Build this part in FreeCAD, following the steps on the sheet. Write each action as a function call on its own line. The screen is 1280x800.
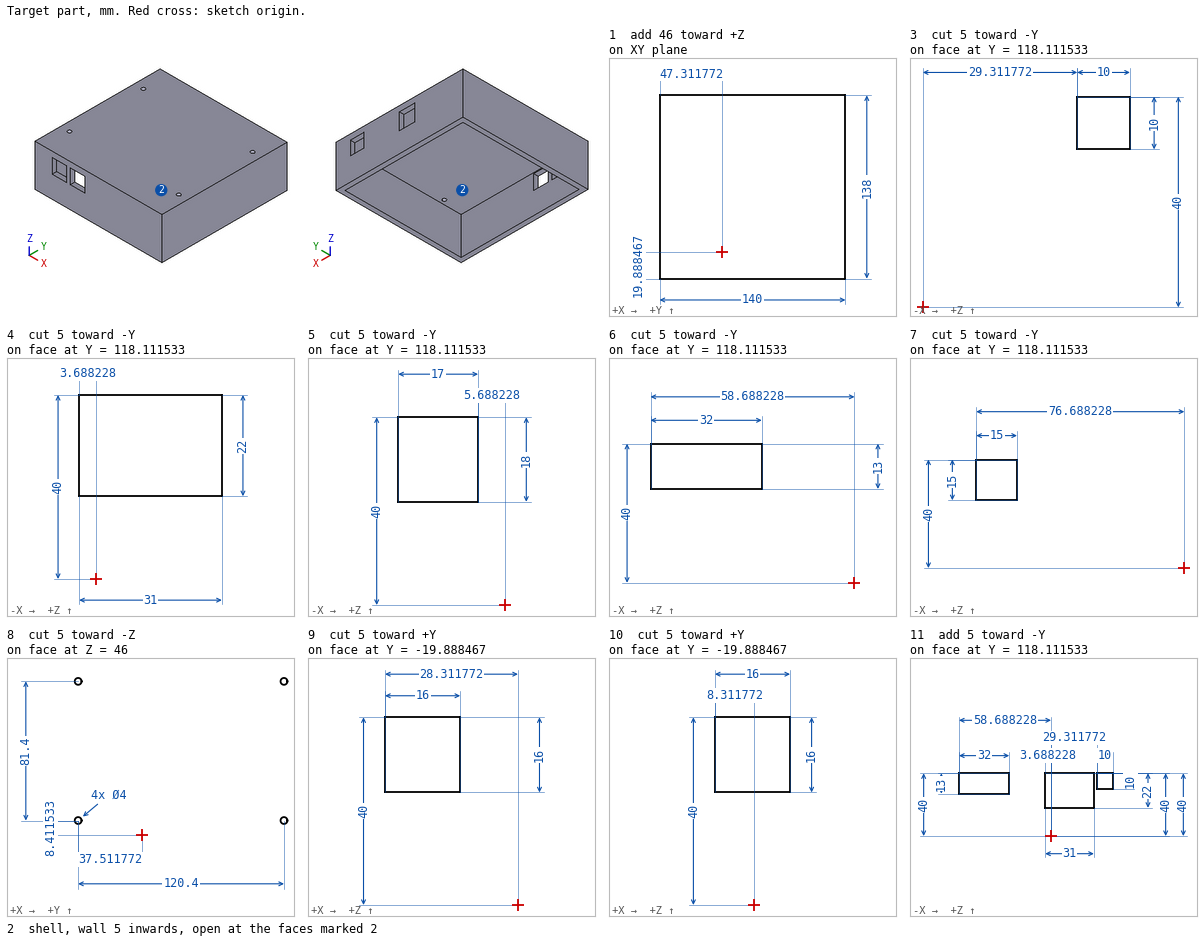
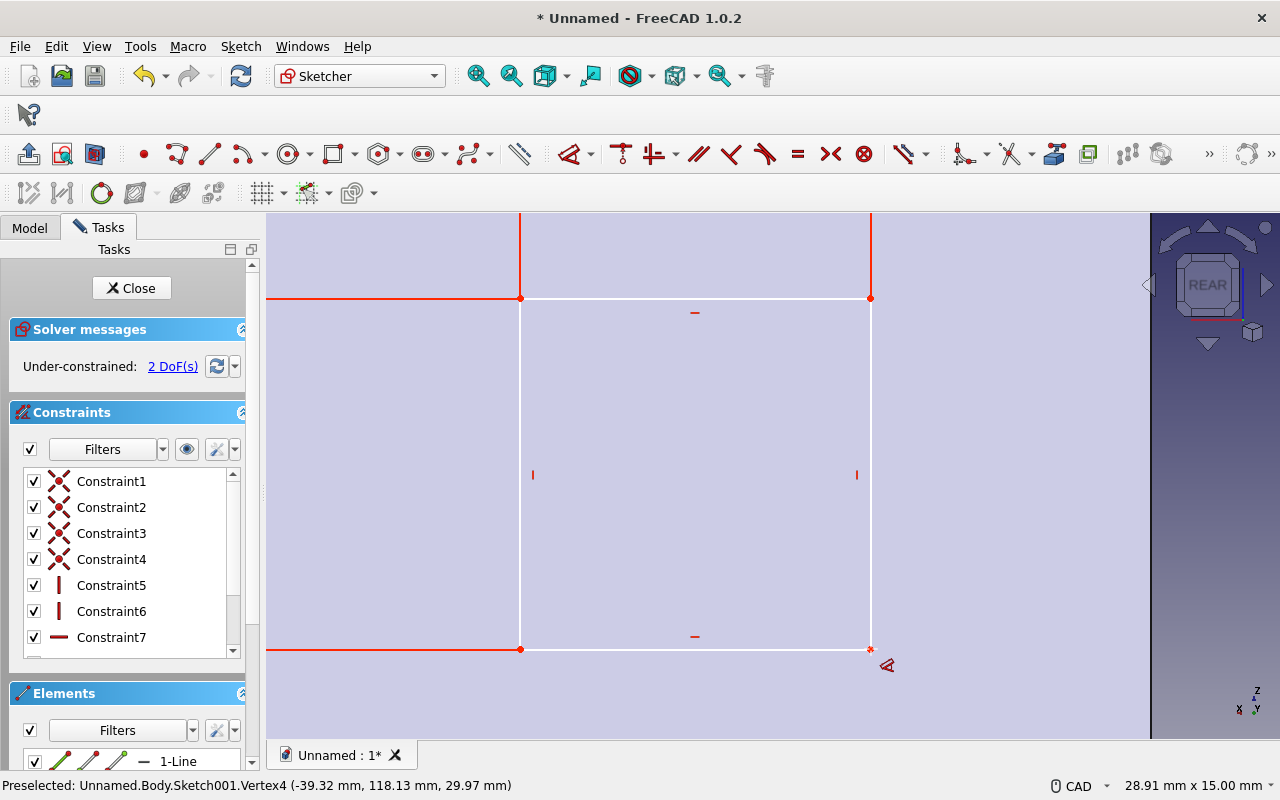
click(520, 299)
click(554, 505)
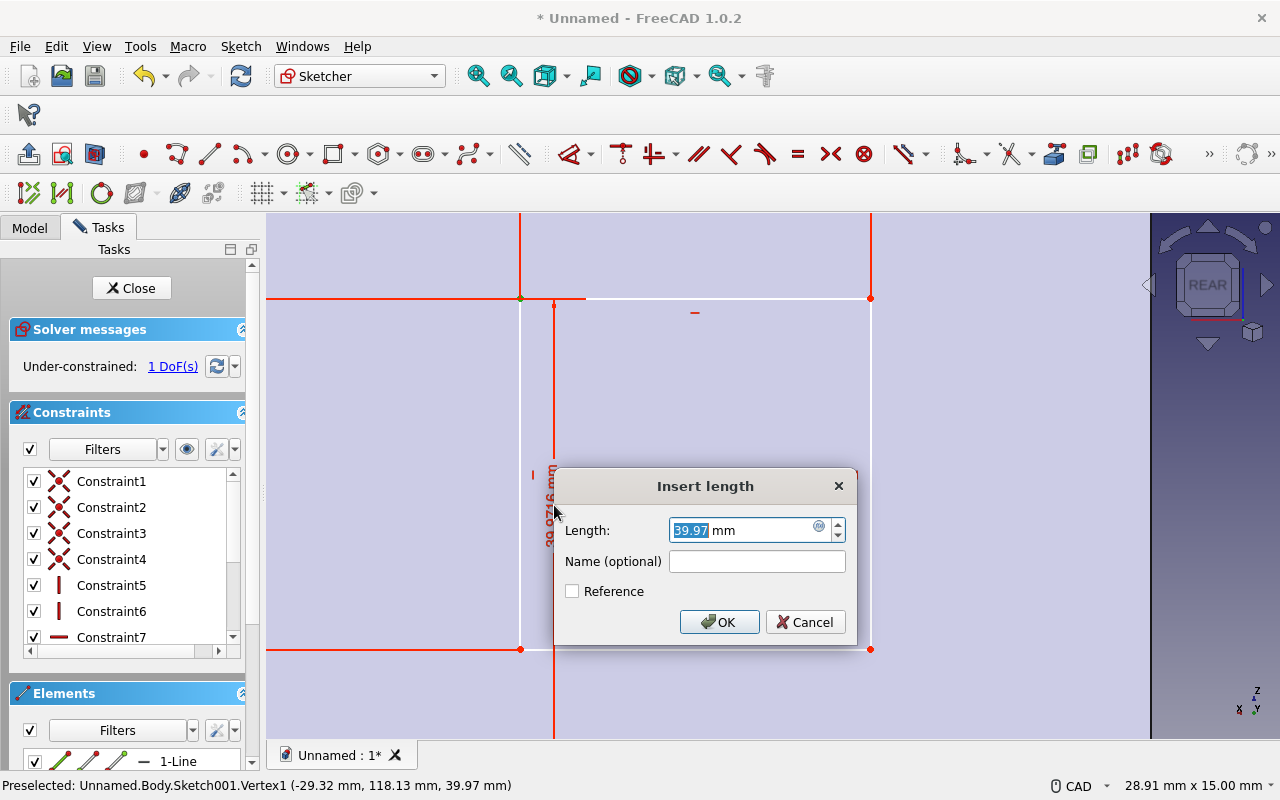
text(40)
key(Return)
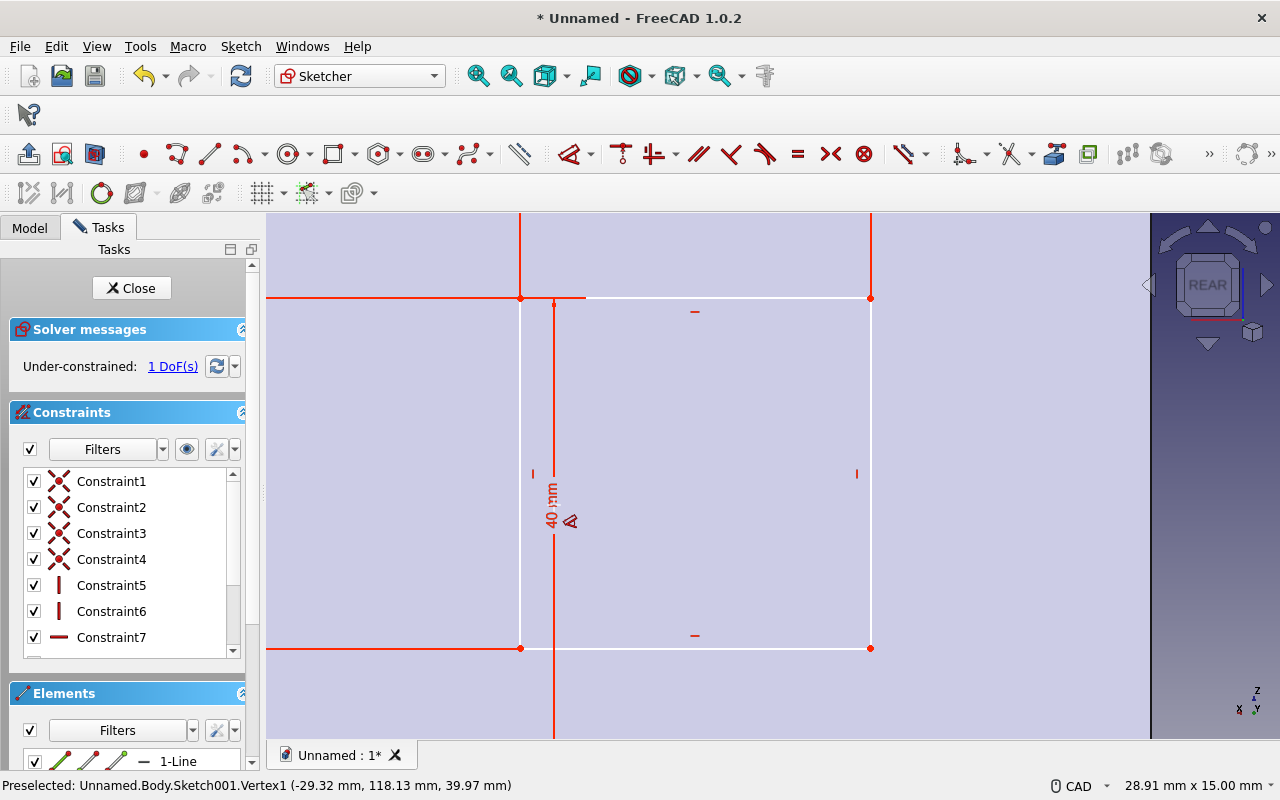
click(520, 298)
click(407, 264)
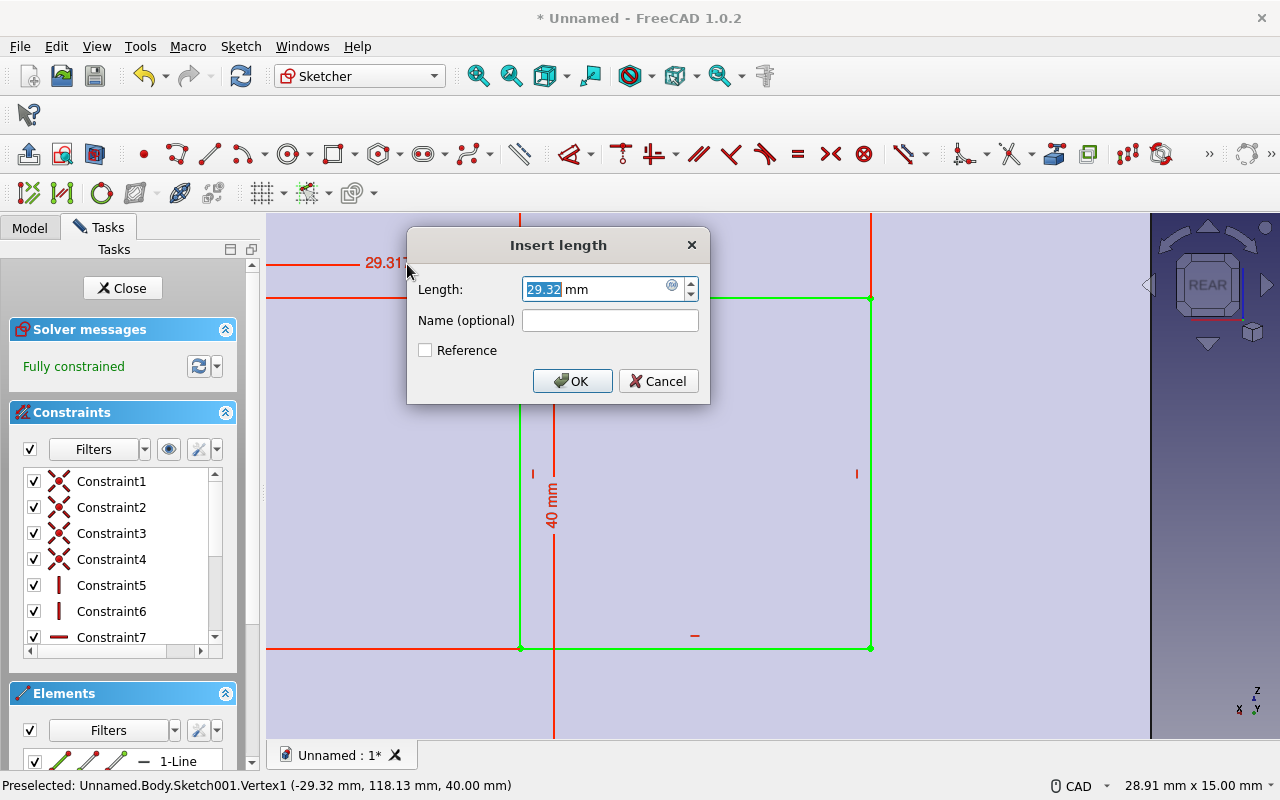
text(29.311772)
key(Return)
key(Escape)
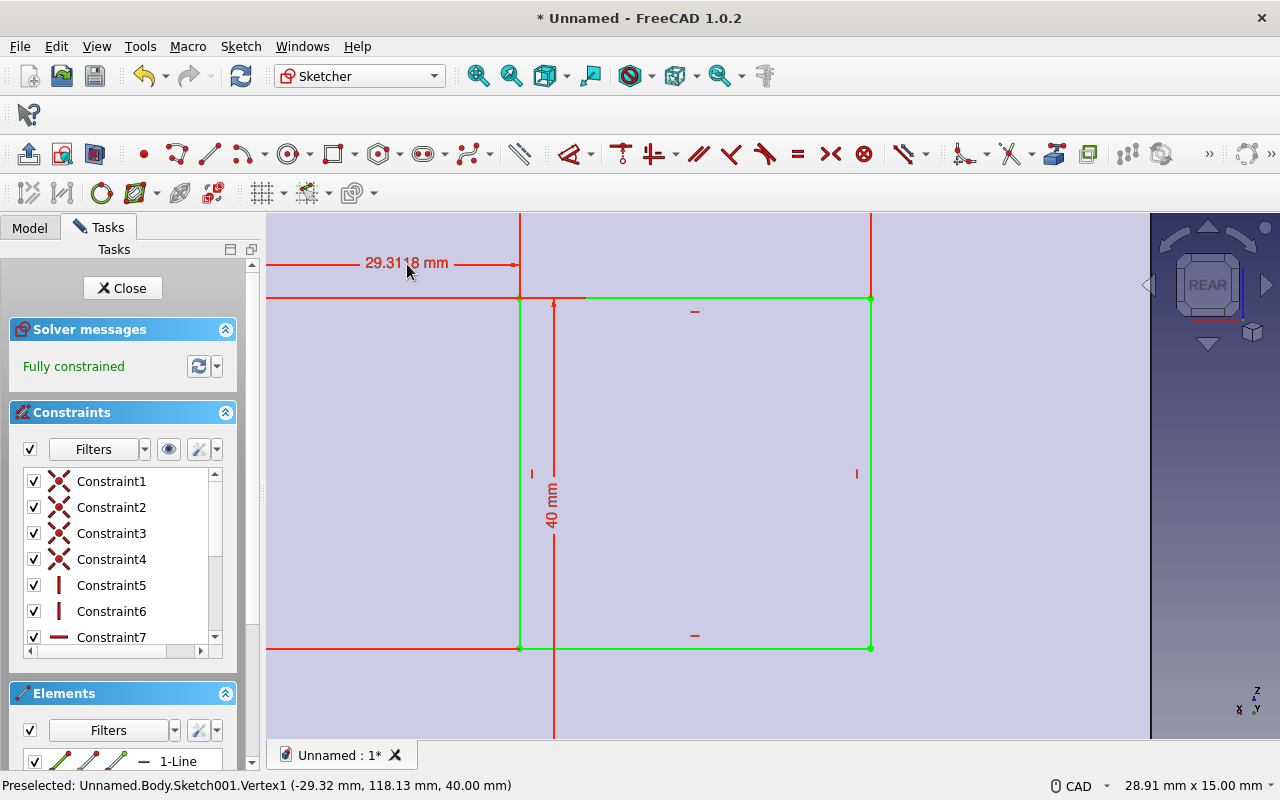
click(123, 288)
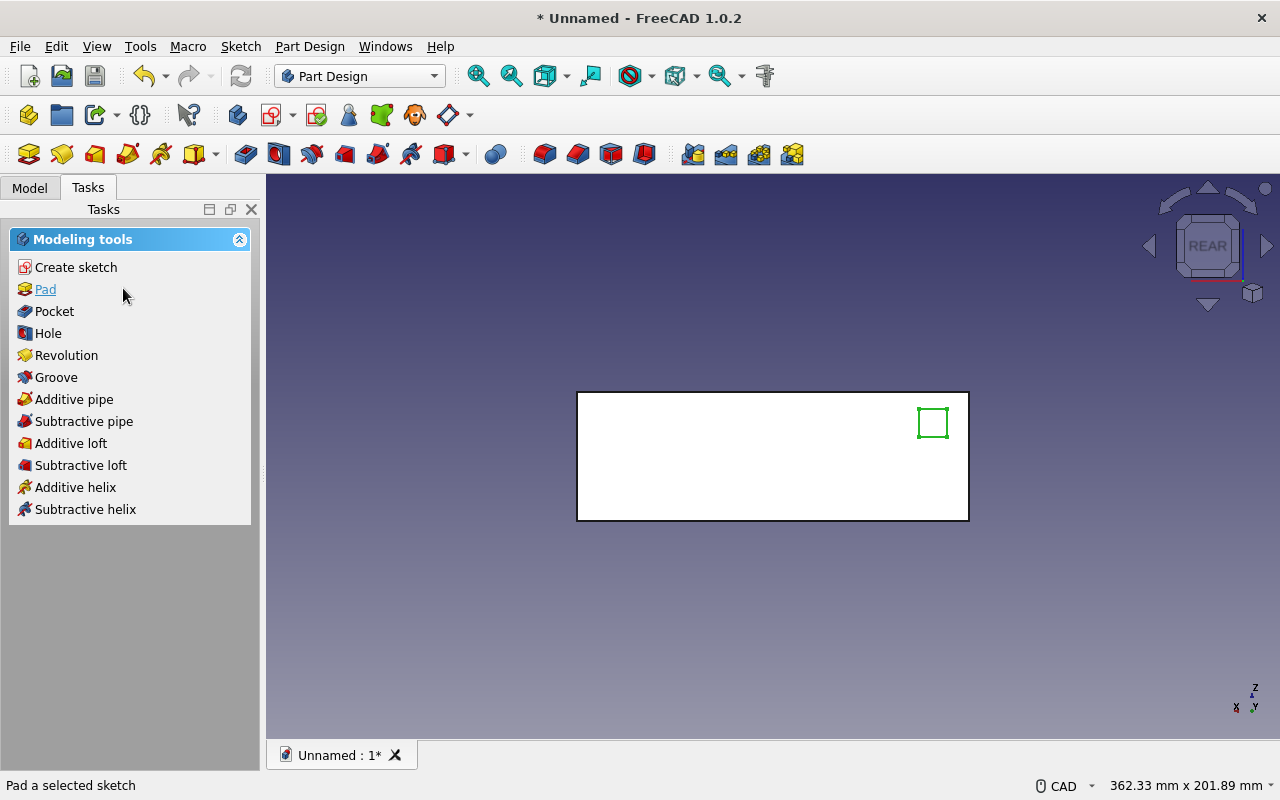
click(246, 154)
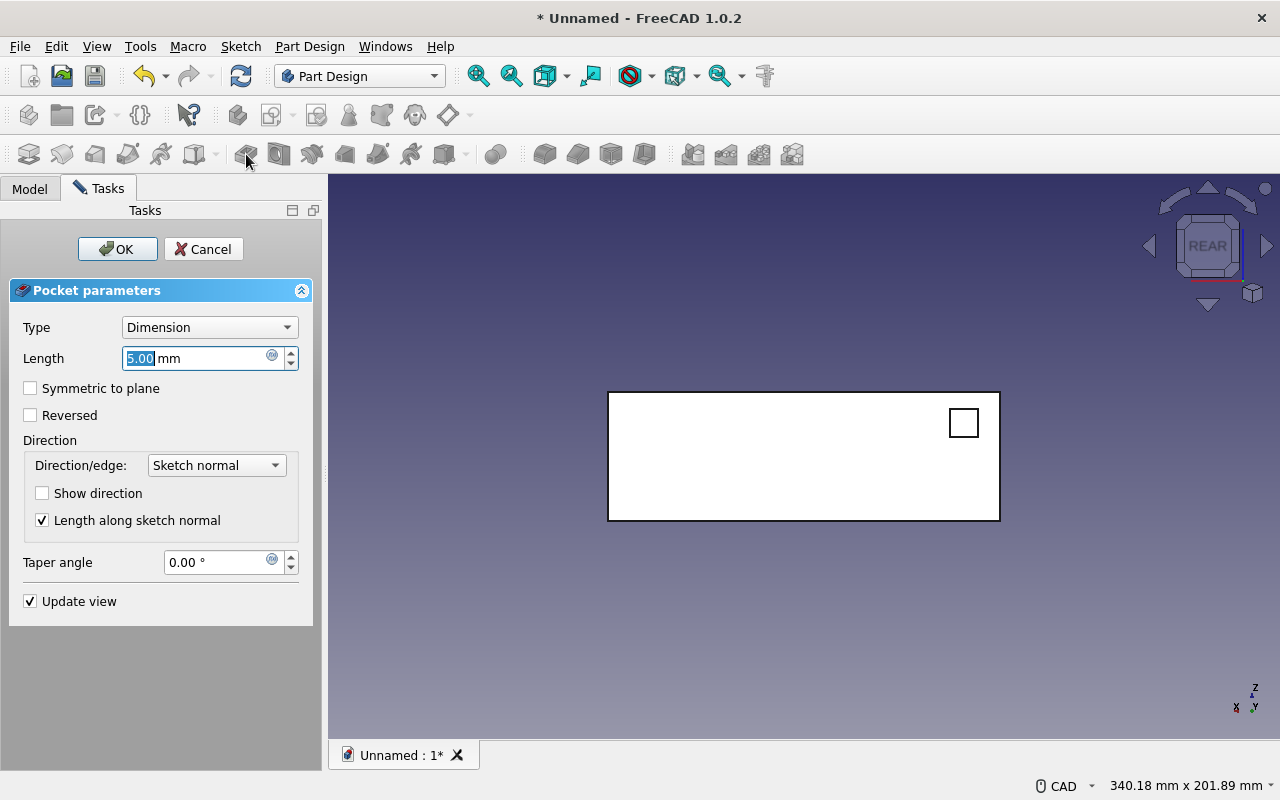
text(5)
key(Tab)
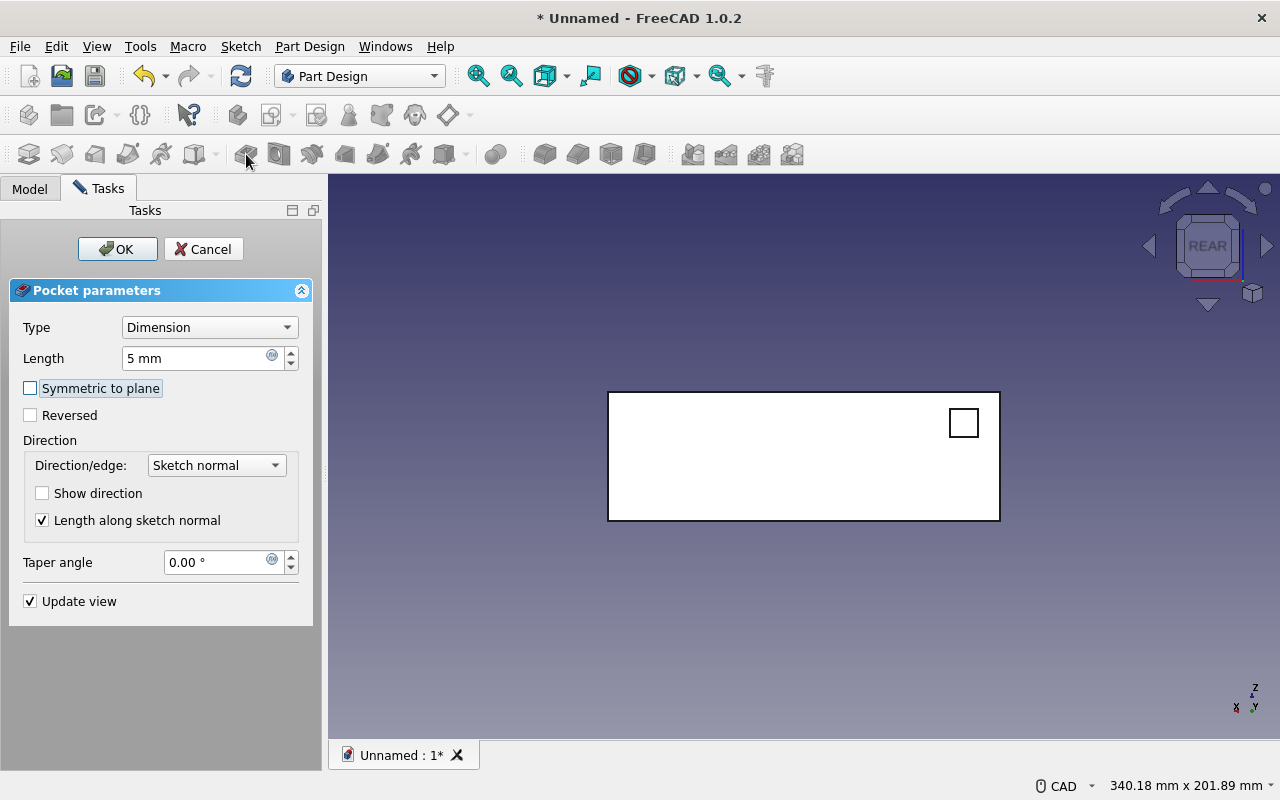
click(118, 249)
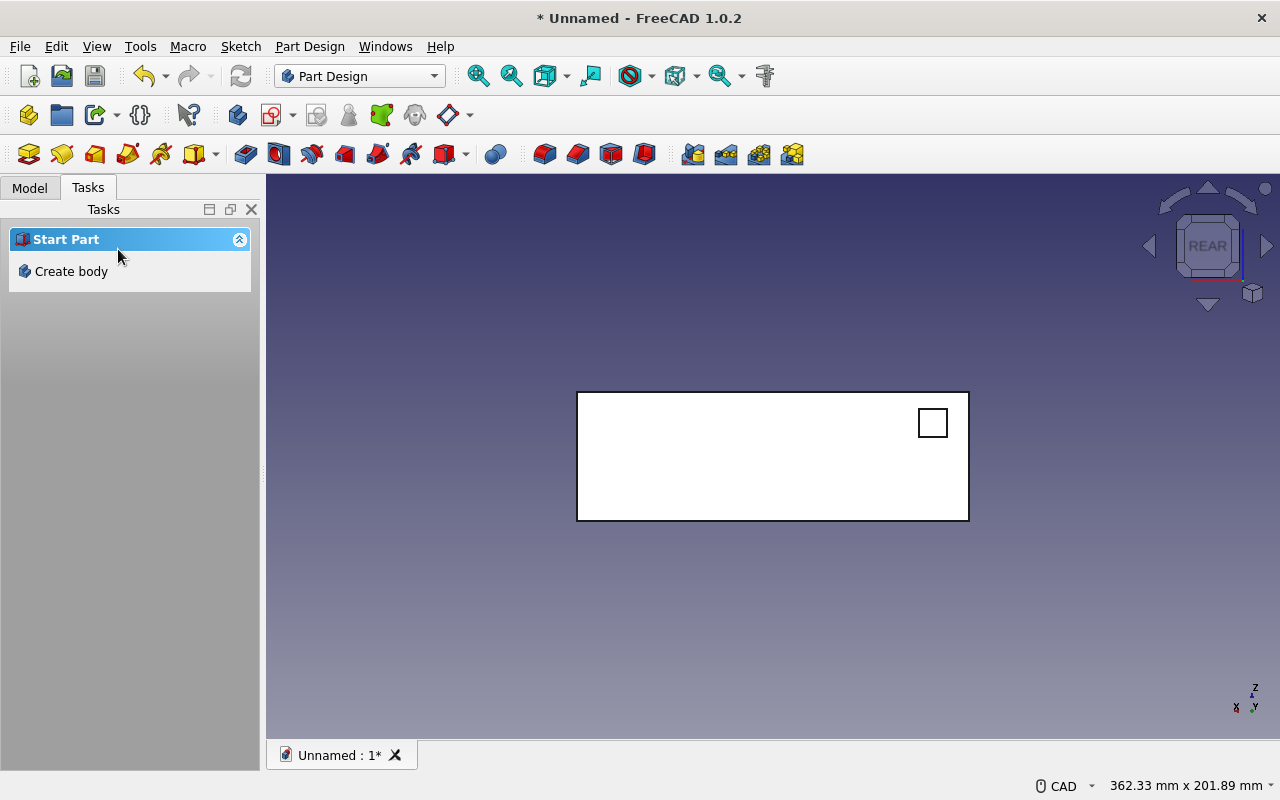
key(v)
key(f)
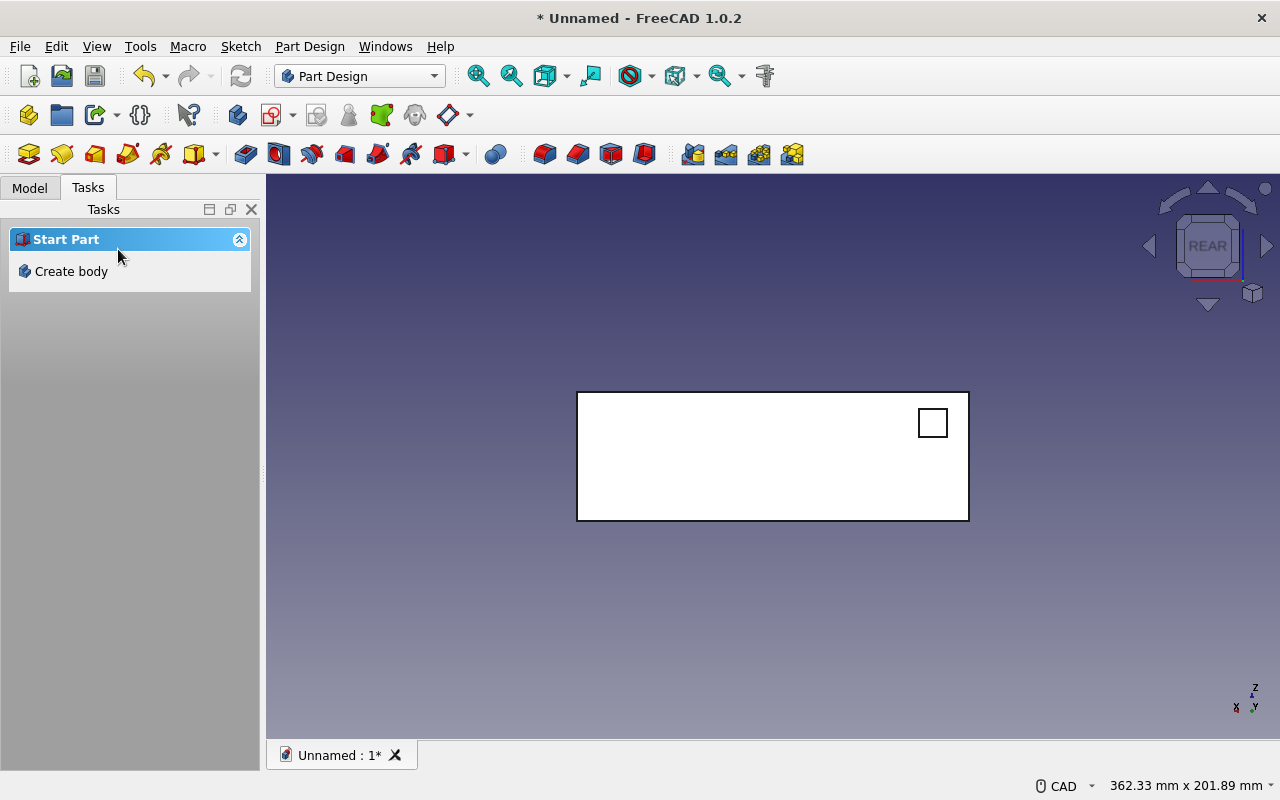
click(661, 455)